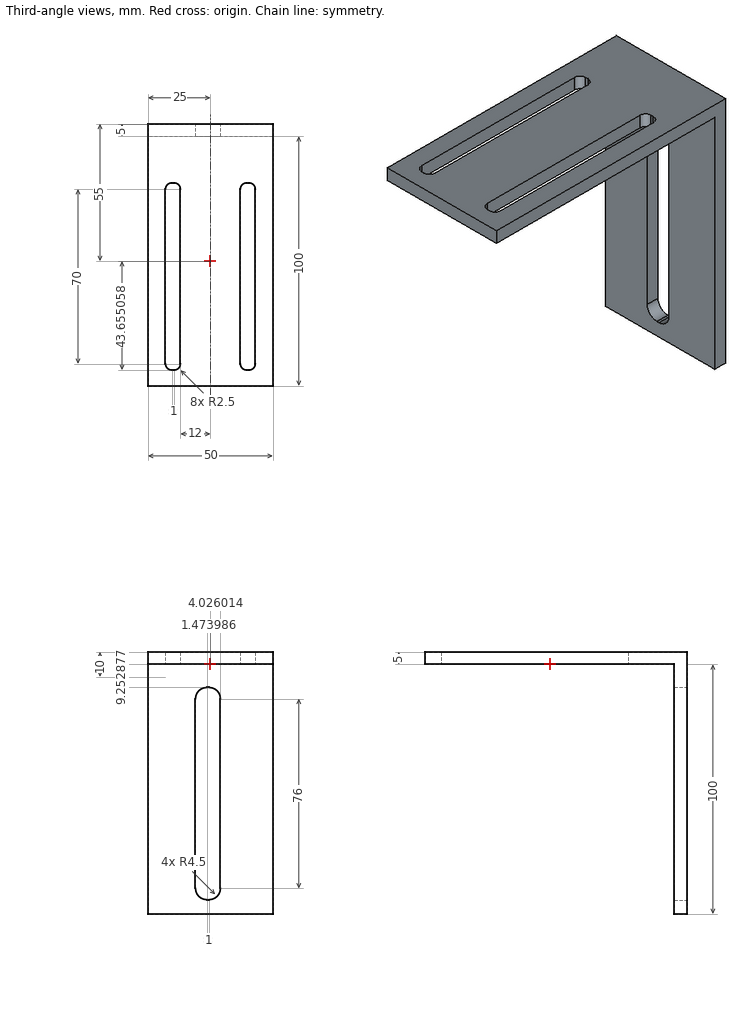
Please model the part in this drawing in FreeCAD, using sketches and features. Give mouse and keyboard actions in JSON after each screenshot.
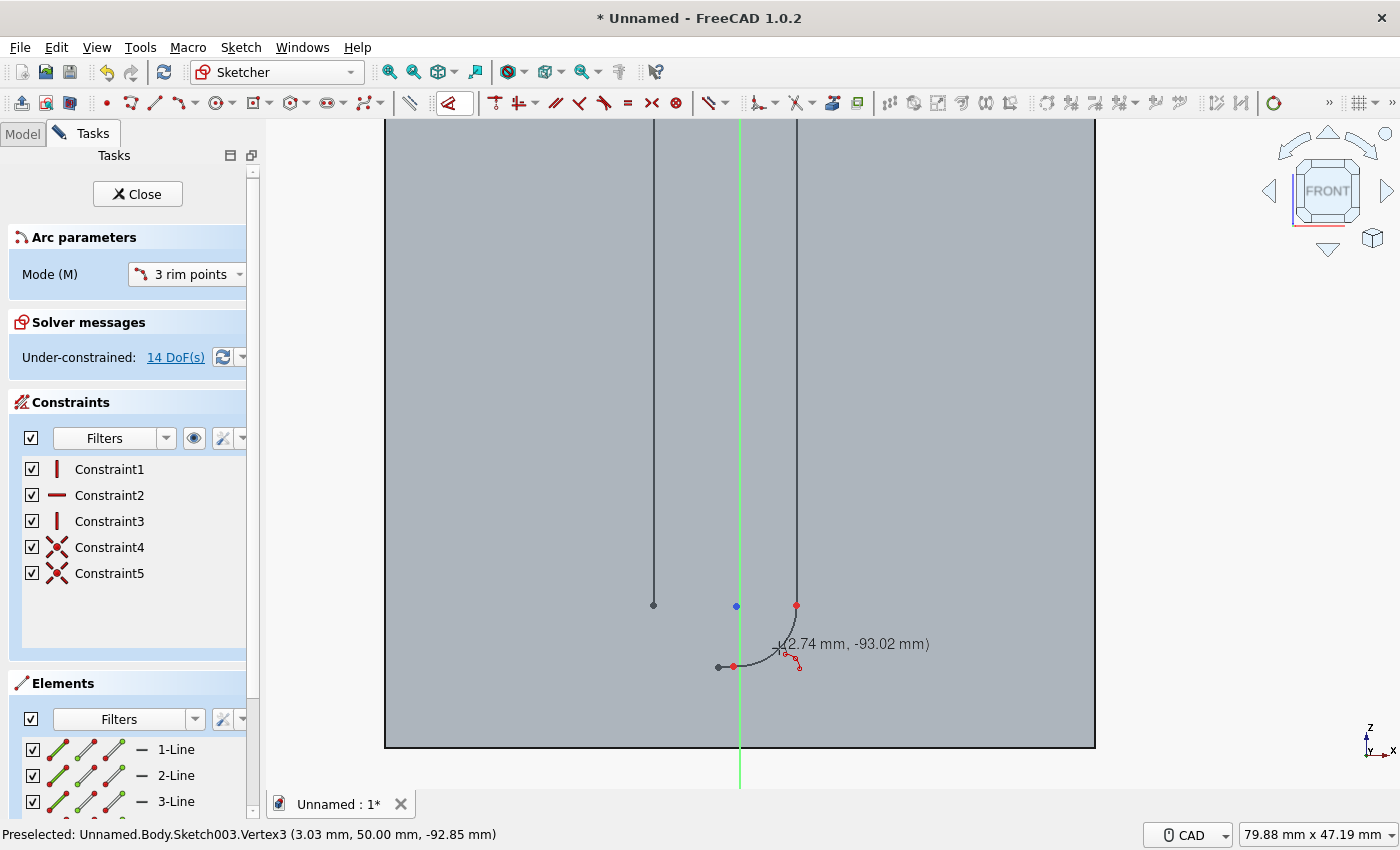
{"action": "scroll", "coordinate": [781, 651], "scroll_direction": "down", "scroll_amount": 6}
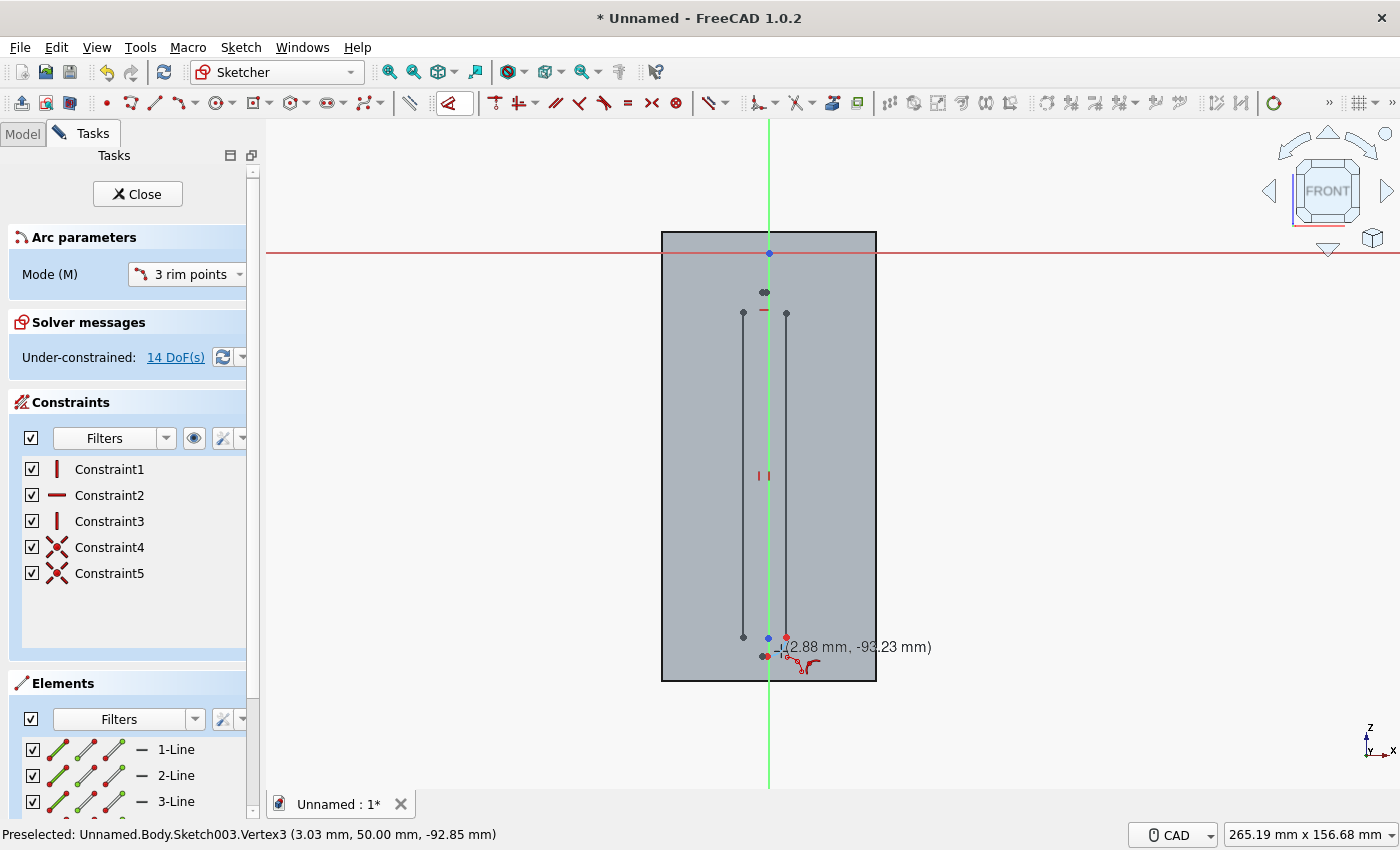
{"action": "left_click", "coordinate": [786, 313]}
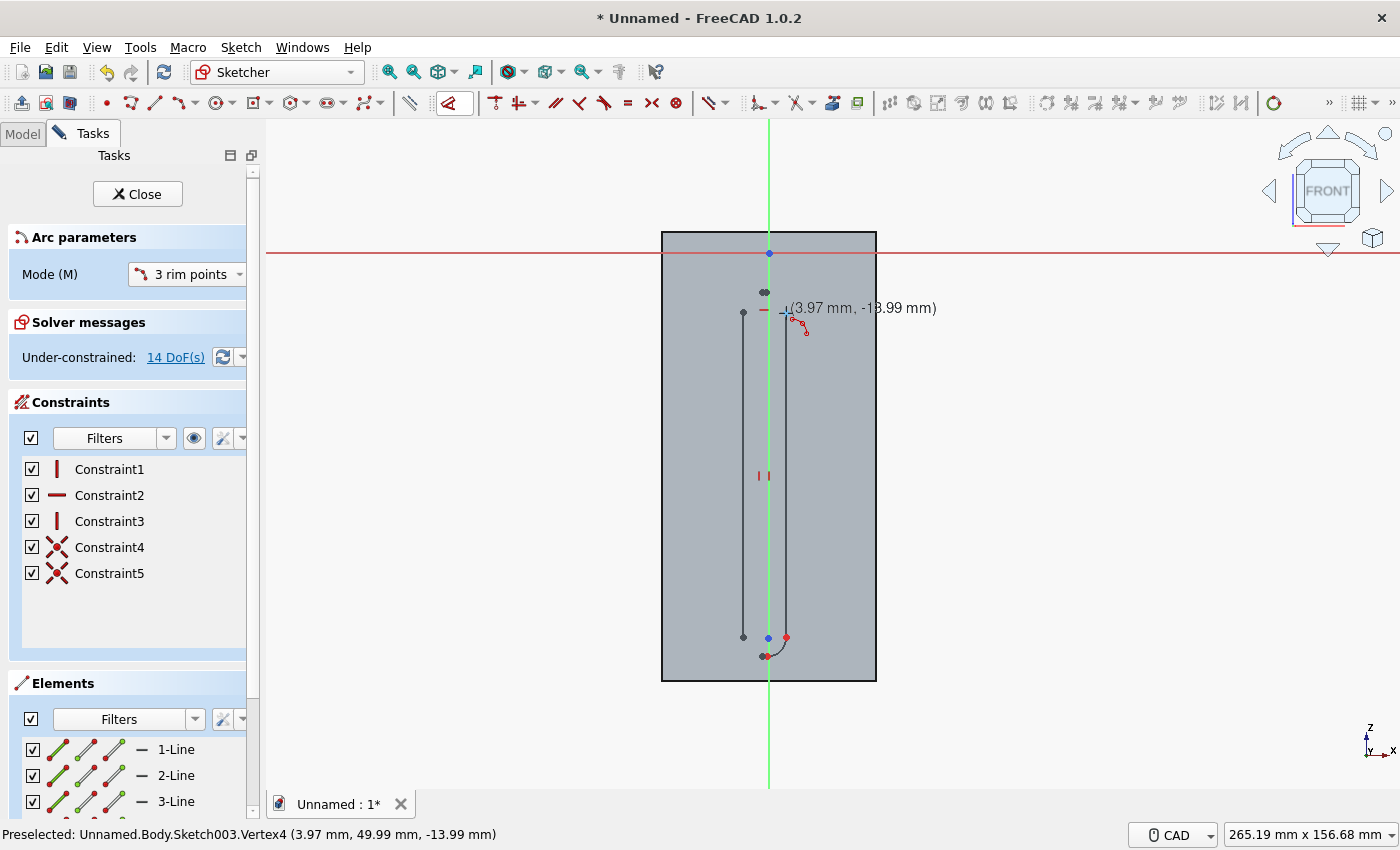
{"action": "scroll", "coordinate": [767, 293], "scroll_direction": "up", "scroll_amount": 11}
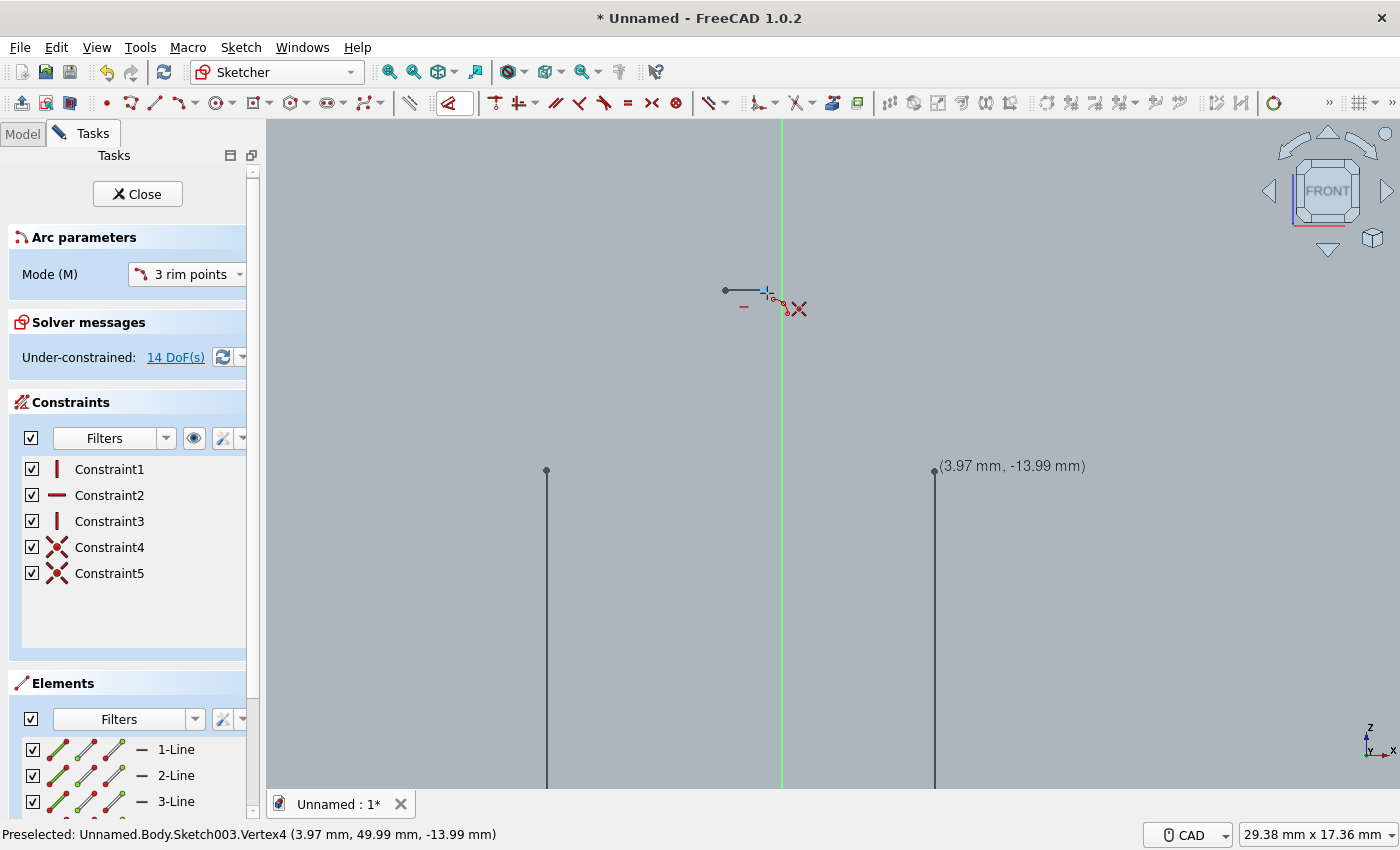
{"action": "left_click", "coordinate": [763, 290]}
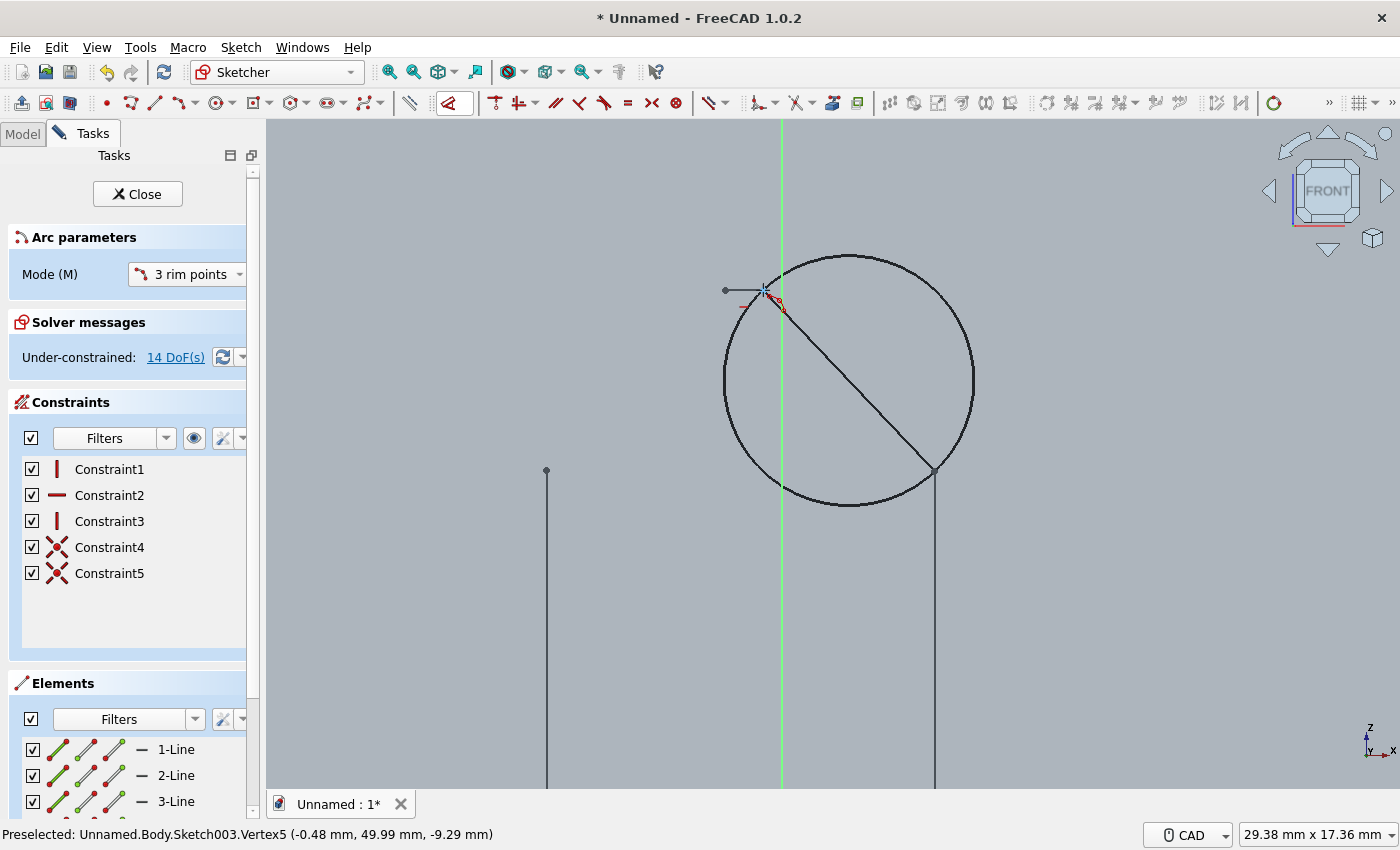
{"action": "scroll", "coordinate": [767, 292], "scroll_direction": "down", "scroll_amount": 11}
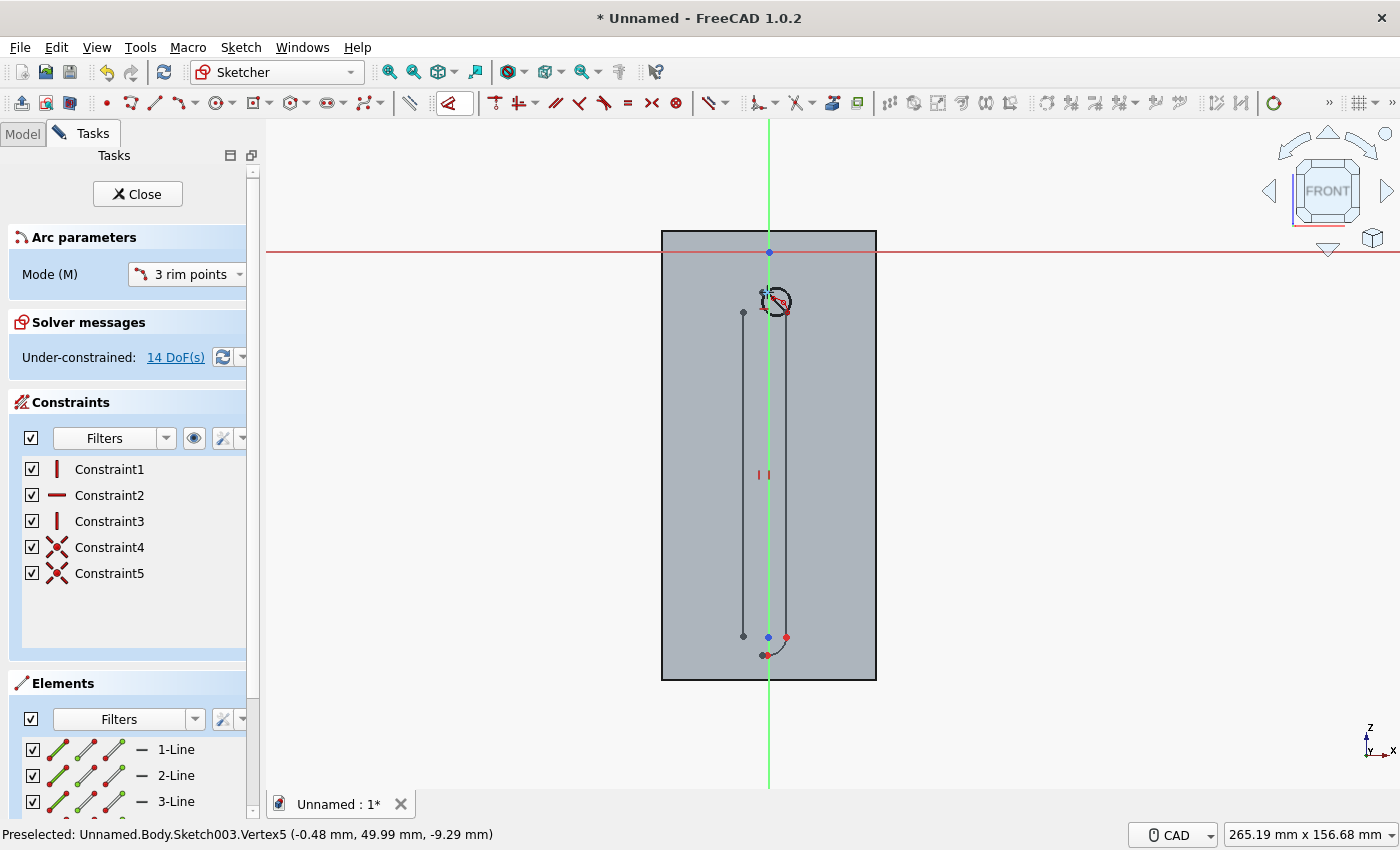
{"action": "scroll", "coordinate": [781, 297], "scroll_direction": "up", "scroll_amount": 6}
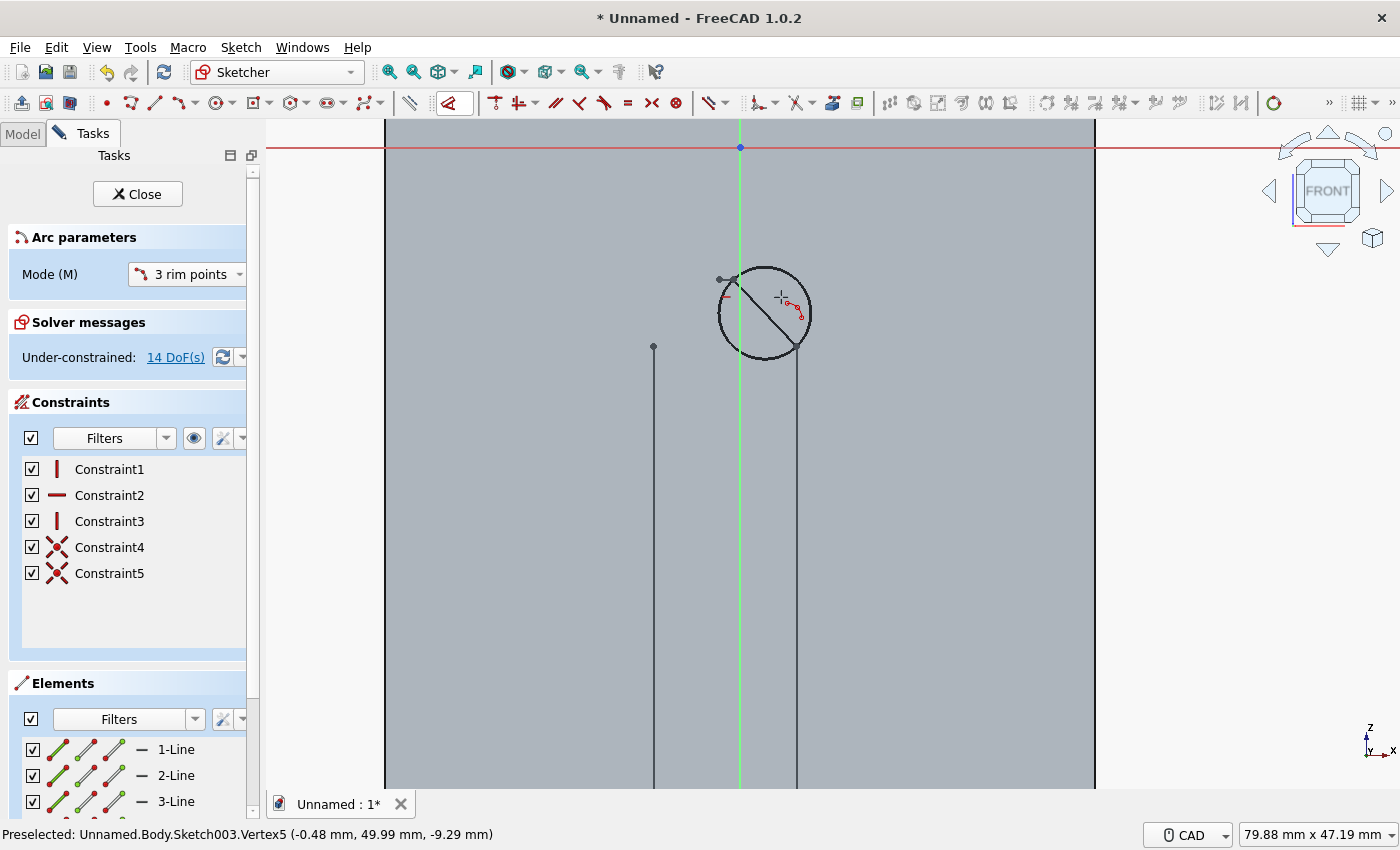
{"action": "left_click", "coordinate": [779, 298]}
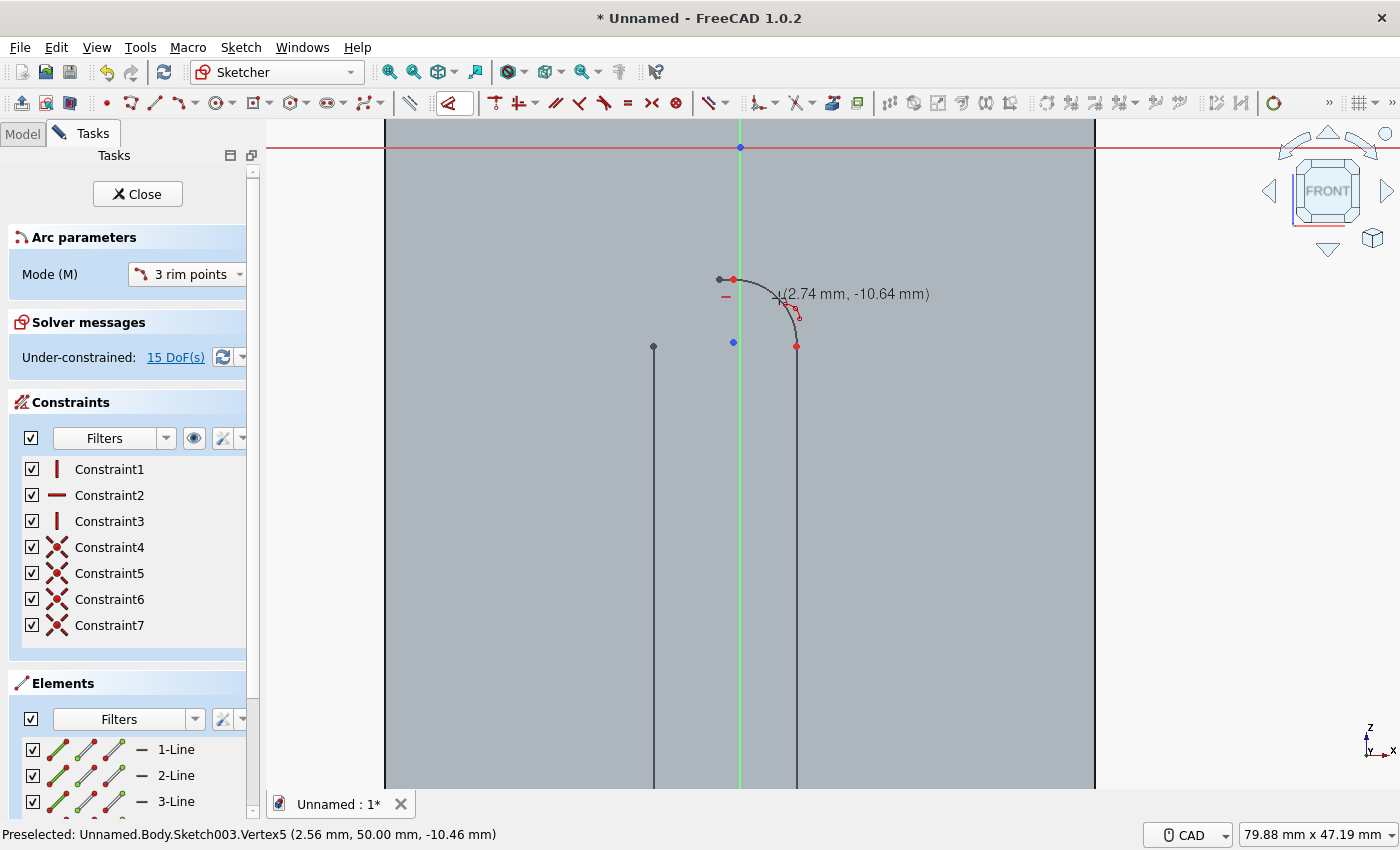
{"action": "scroll", "coordinate": [719, 279], "scroll_direction": "up", "scroll_amount": 5}